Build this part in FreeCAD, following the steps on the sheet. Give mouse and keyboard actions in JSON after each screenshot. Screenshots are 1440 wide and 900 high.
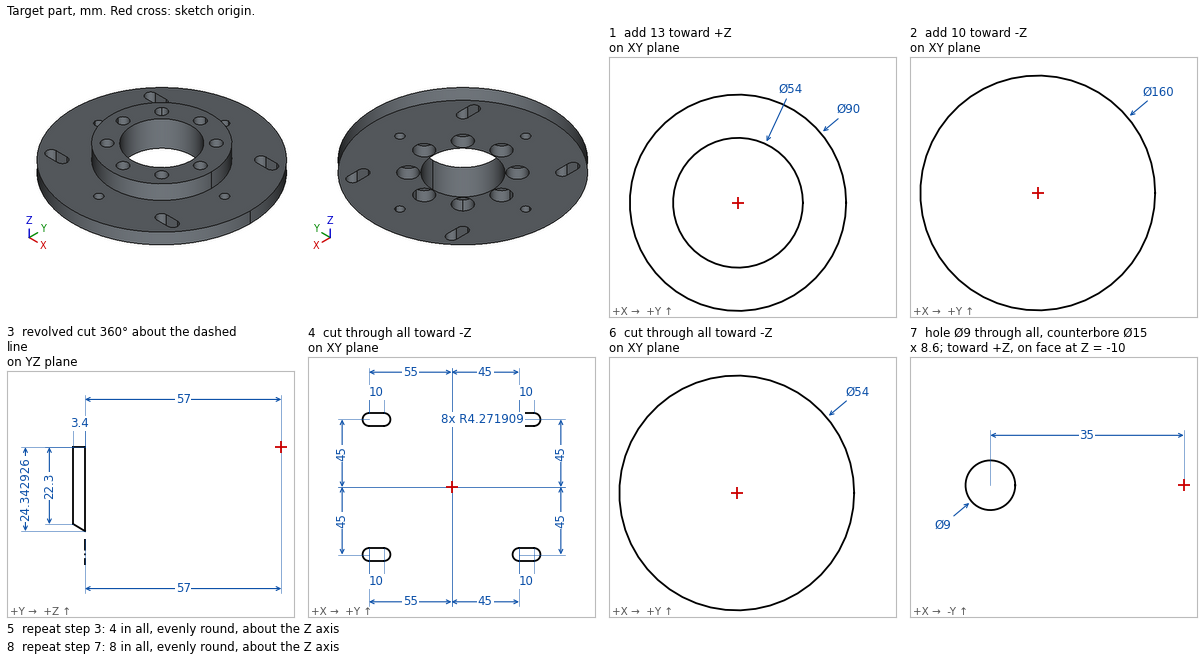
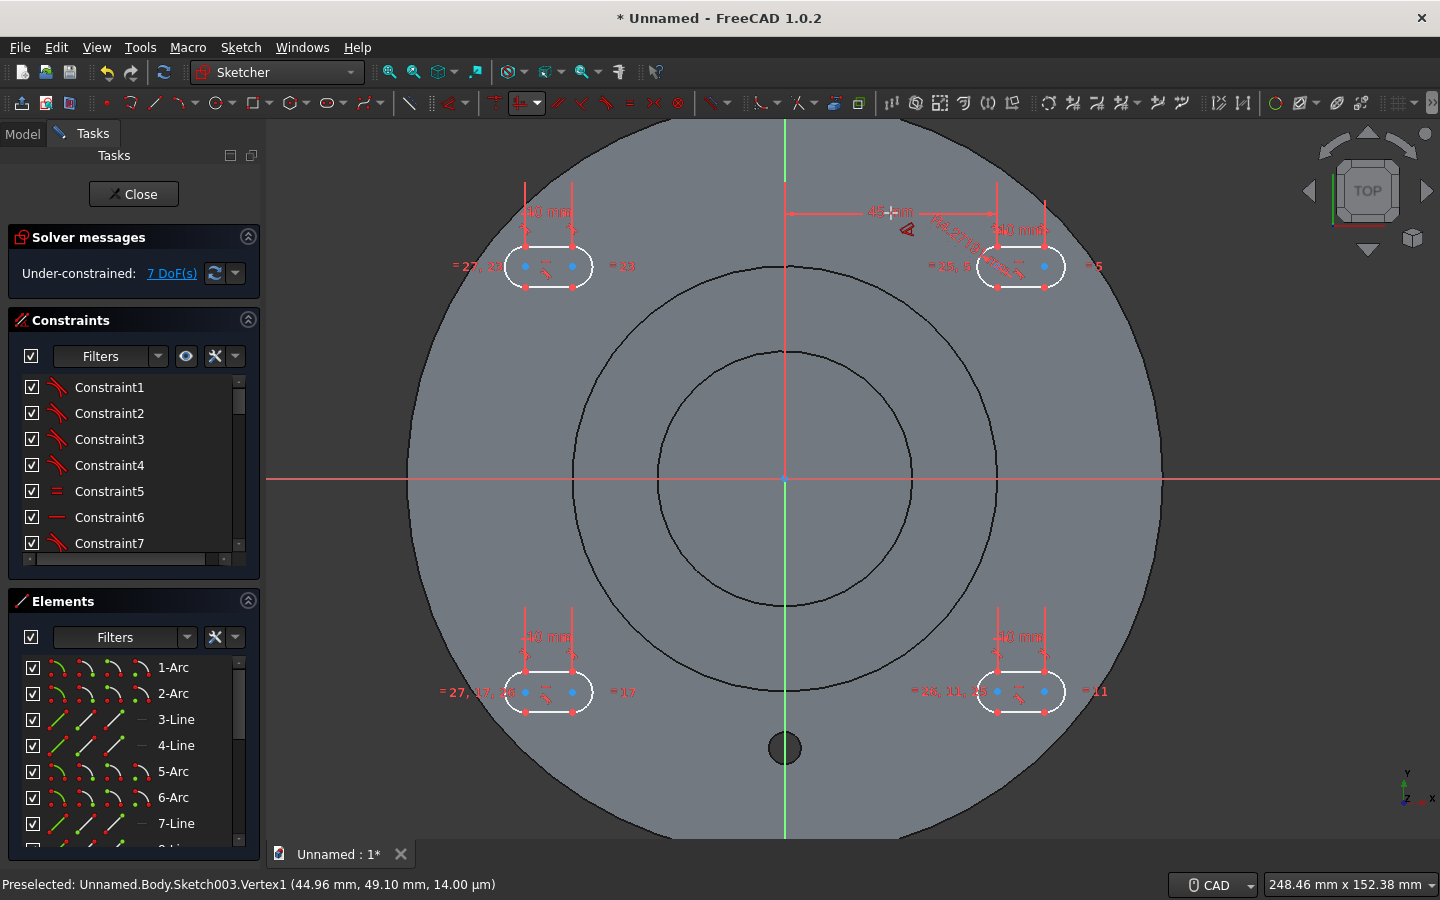
{"action": "left_click", "coordinate": [998, 672]}
{"action": "left_click", "coordinate": [891, 706]}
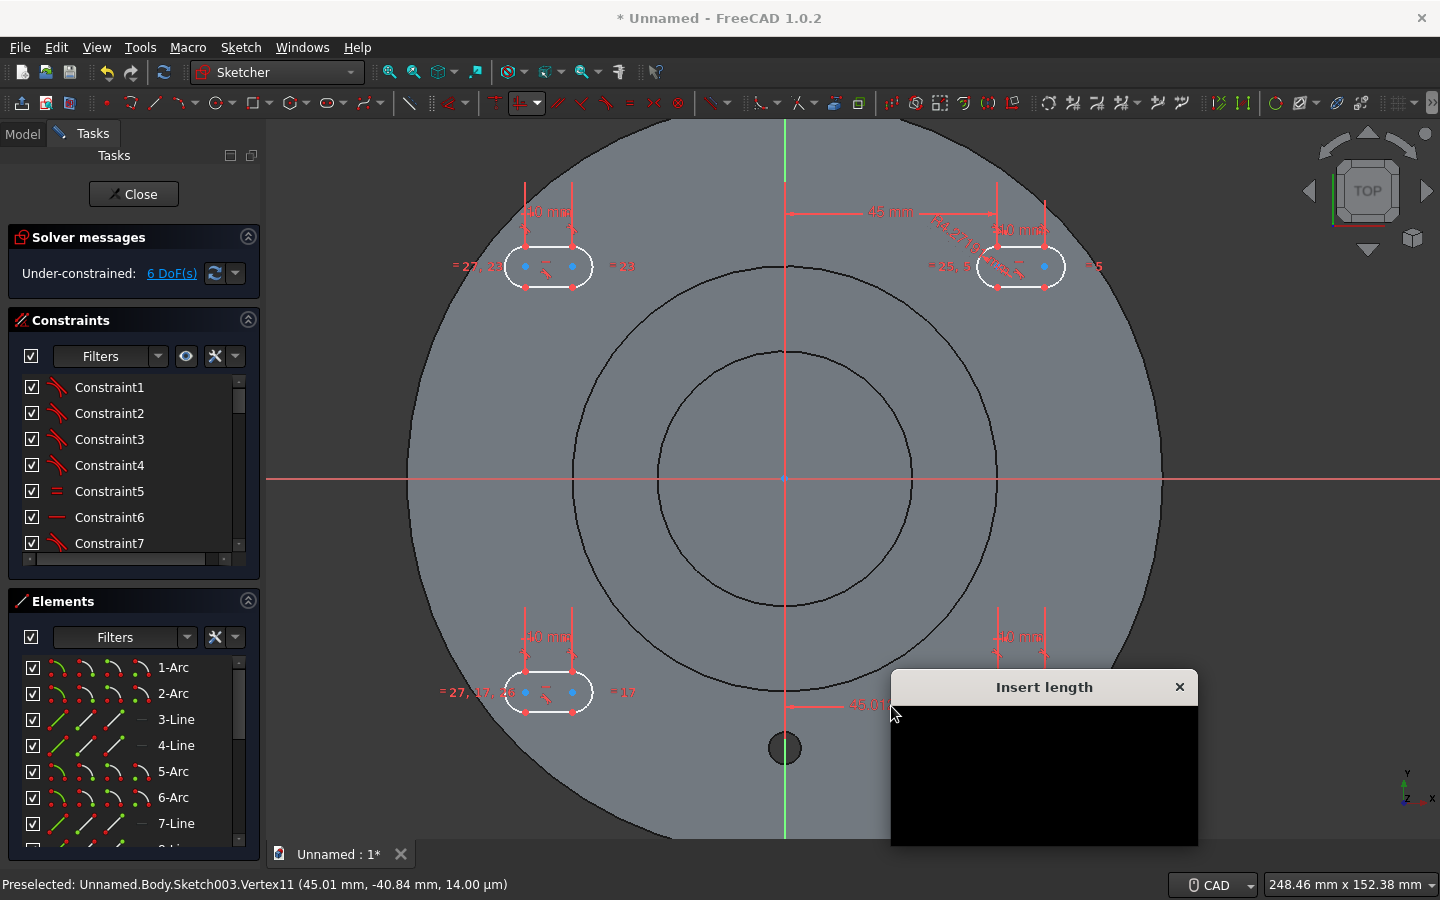
{"action": "type", "text": "45"}
{"action": "key", "text": "Return"}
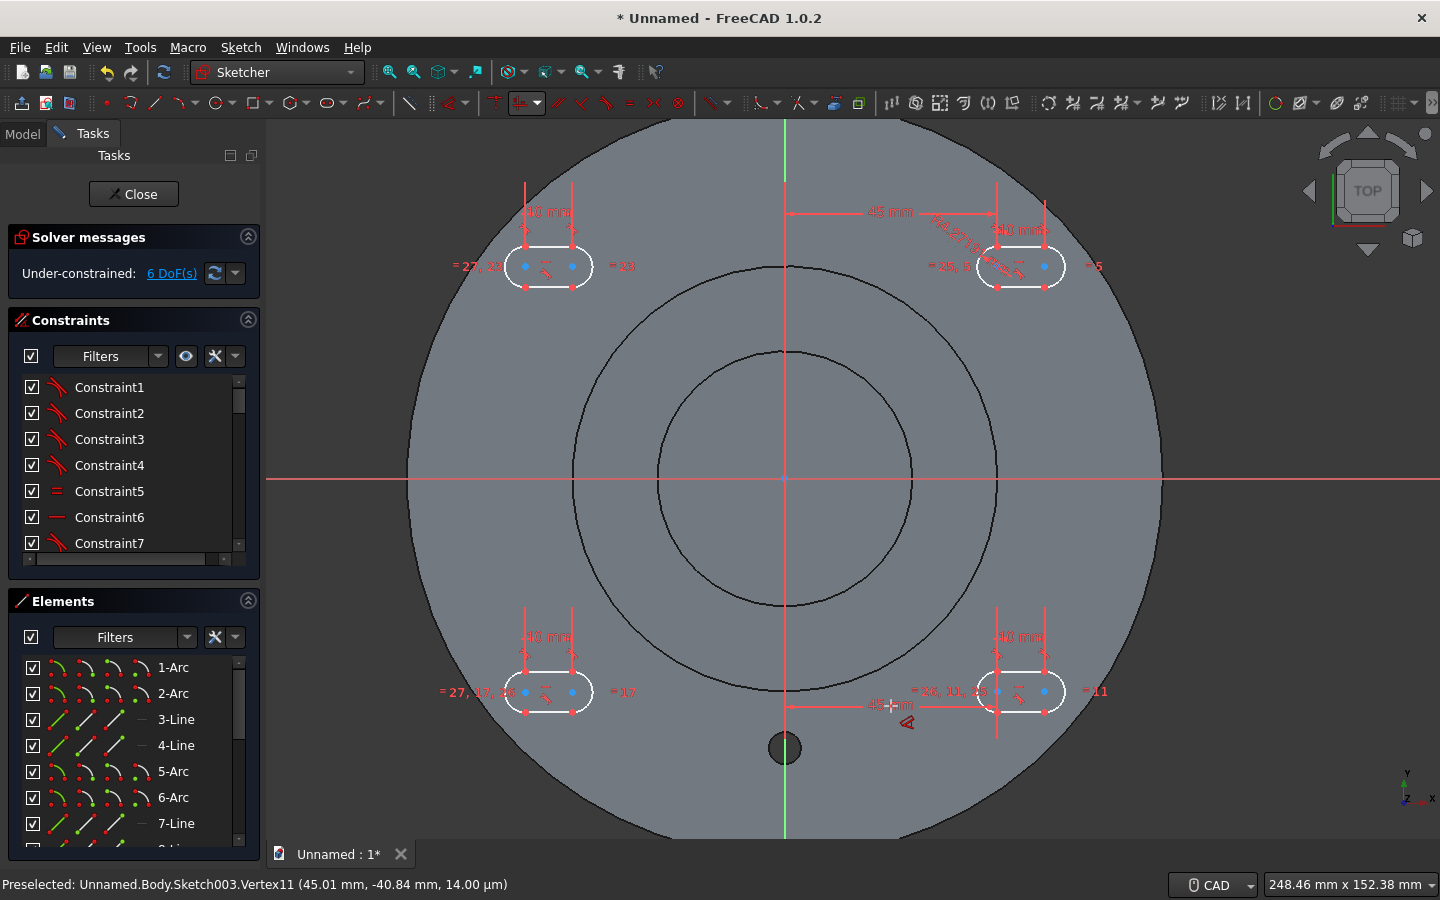
{"action": "left_click", "coordinate": [525, 672]}
{"action": "left_click", "coordinate": [655, 706]}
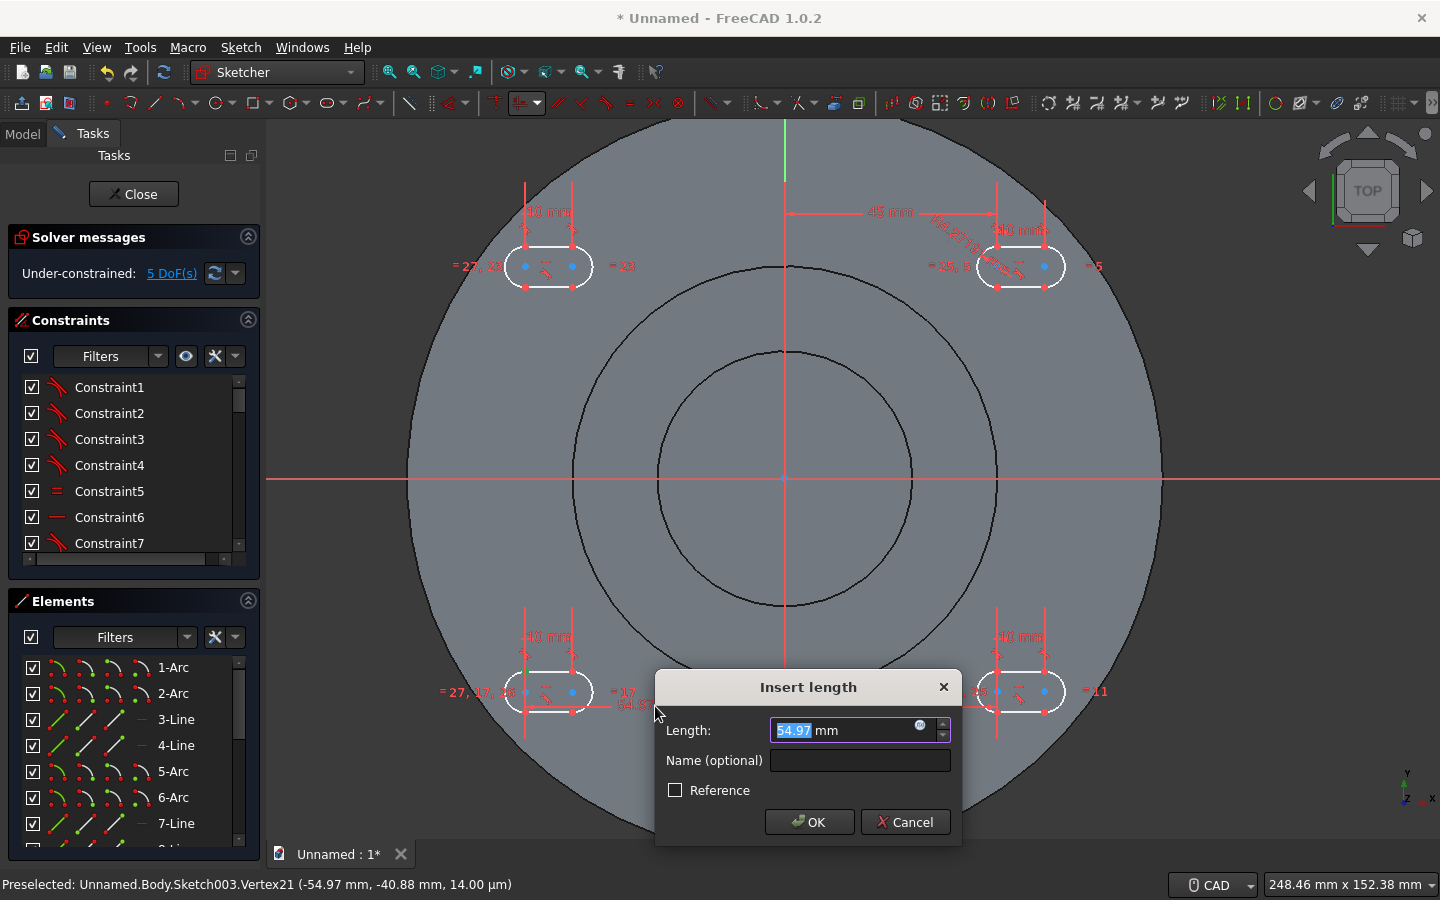
{"action": "type", "text": "55"}
{"action": "key", "text": "Return"}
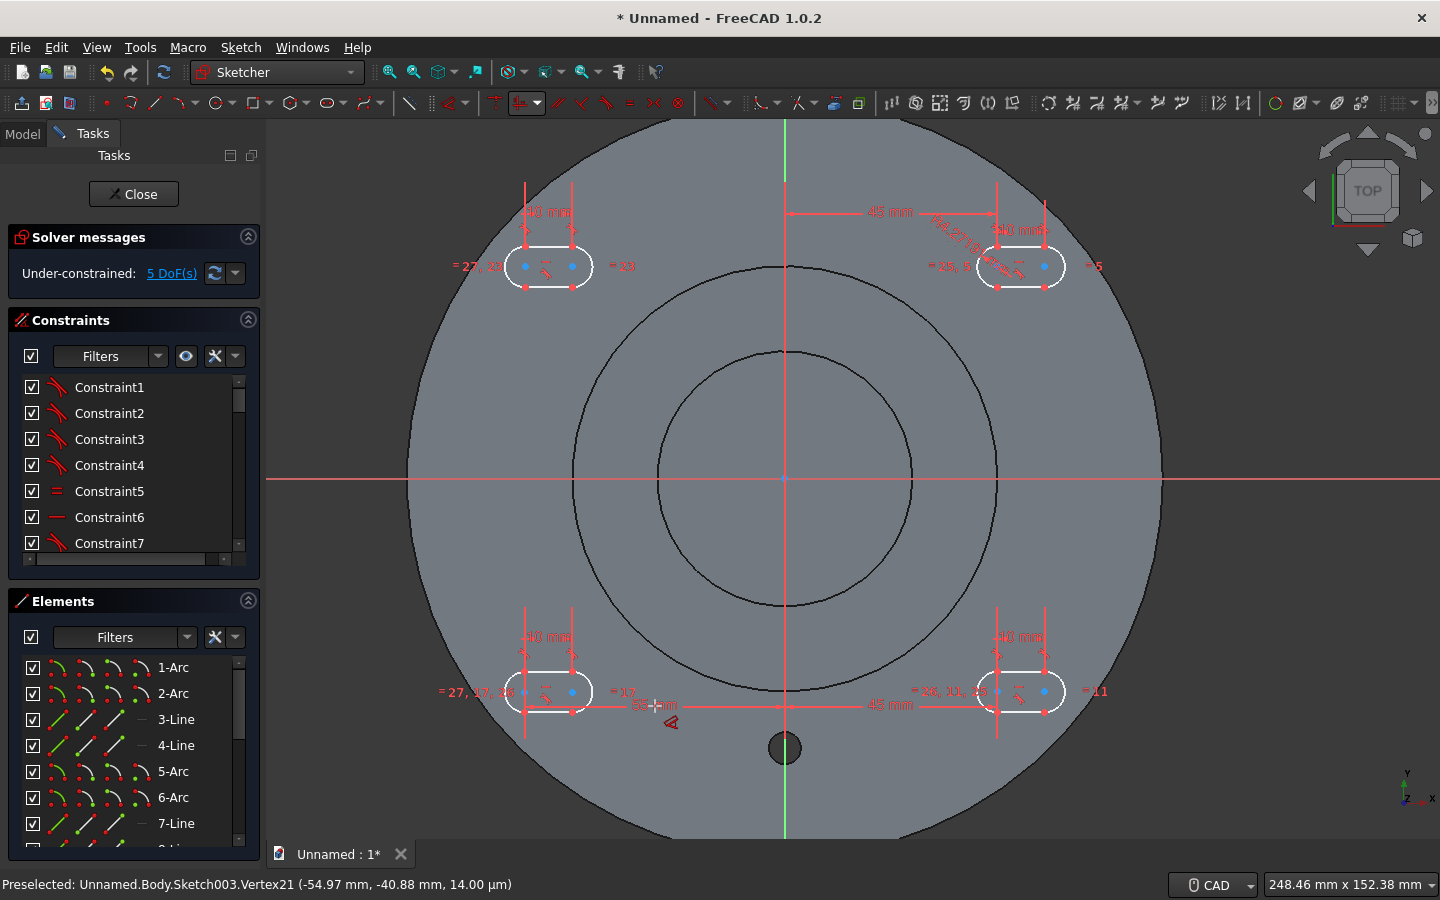
{"action": "left_click", "coordinate": [525, 247]}
{"action": "left_click", "coordinate": [655, 213]}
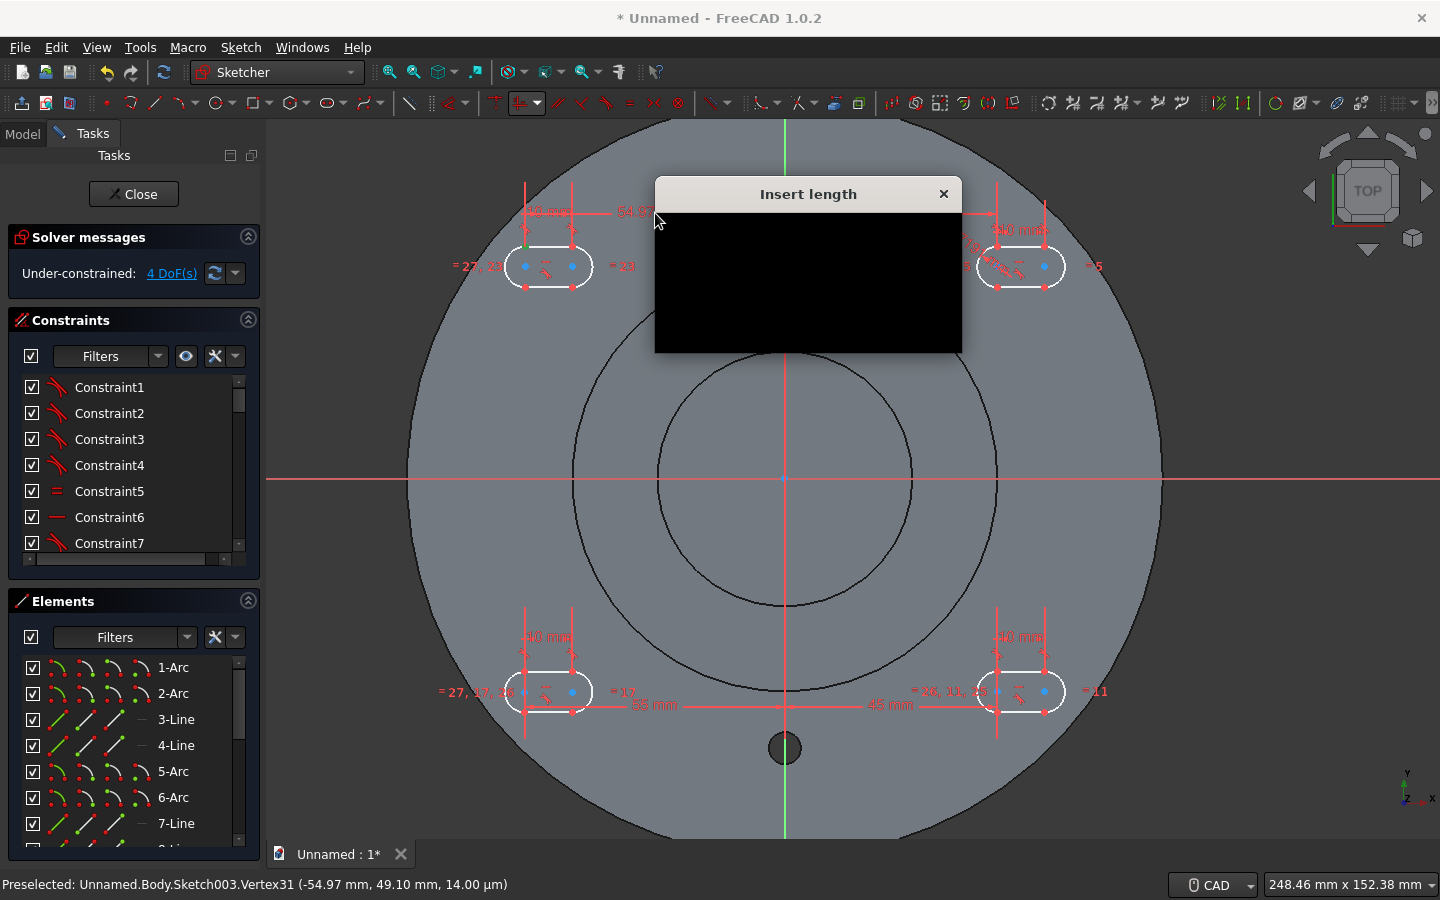
{"action": "type", "text": "55"}
{"action": "key", "text": "Return"}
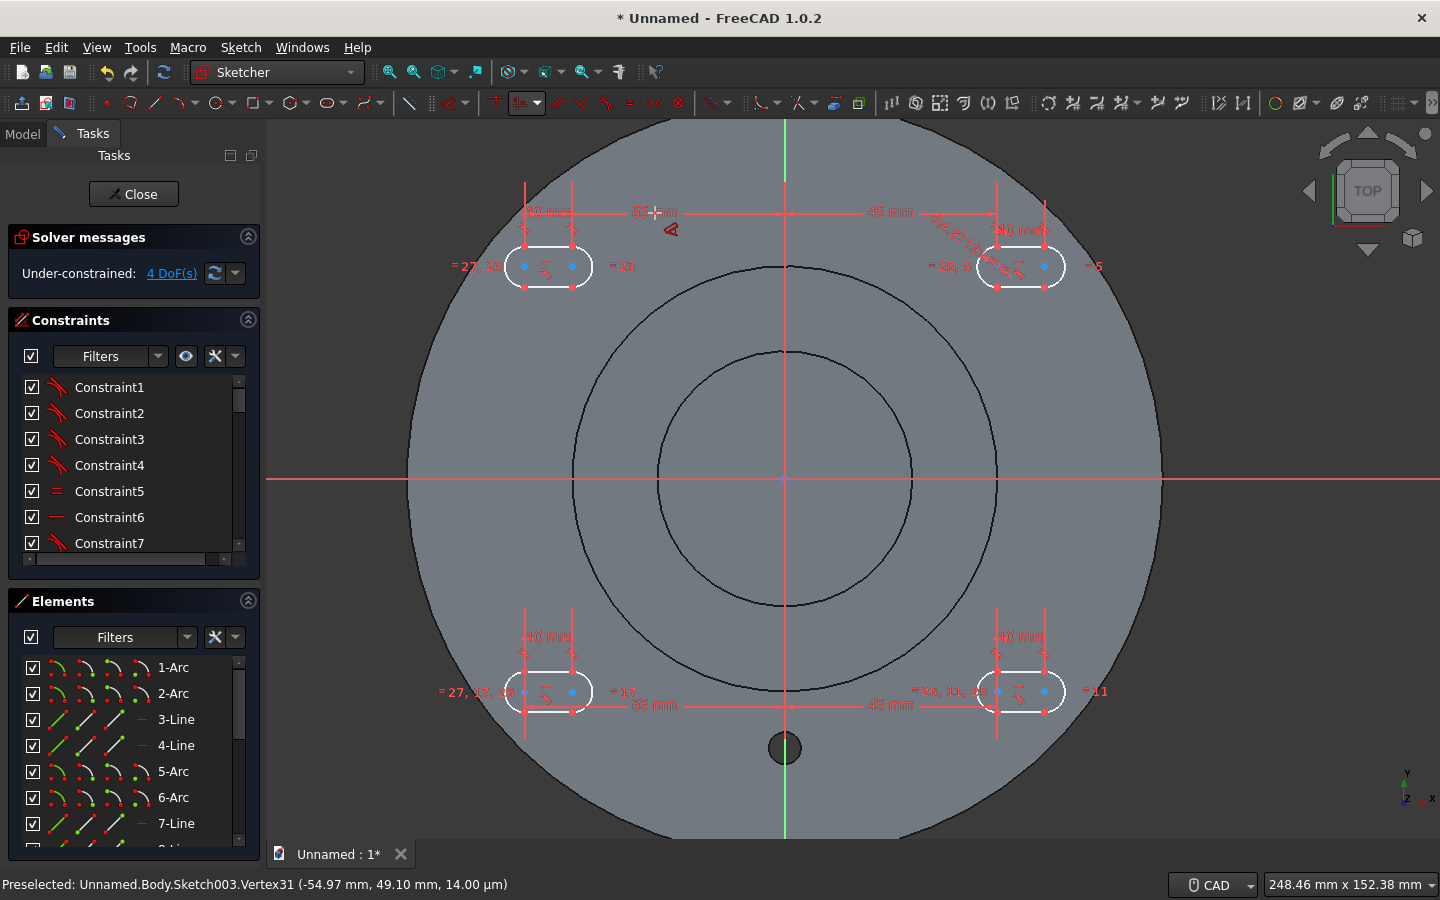
{"action": "left_click", "coordinate": [997, 267]}
{"action": "left_click", "coordinate": [1031, 373]}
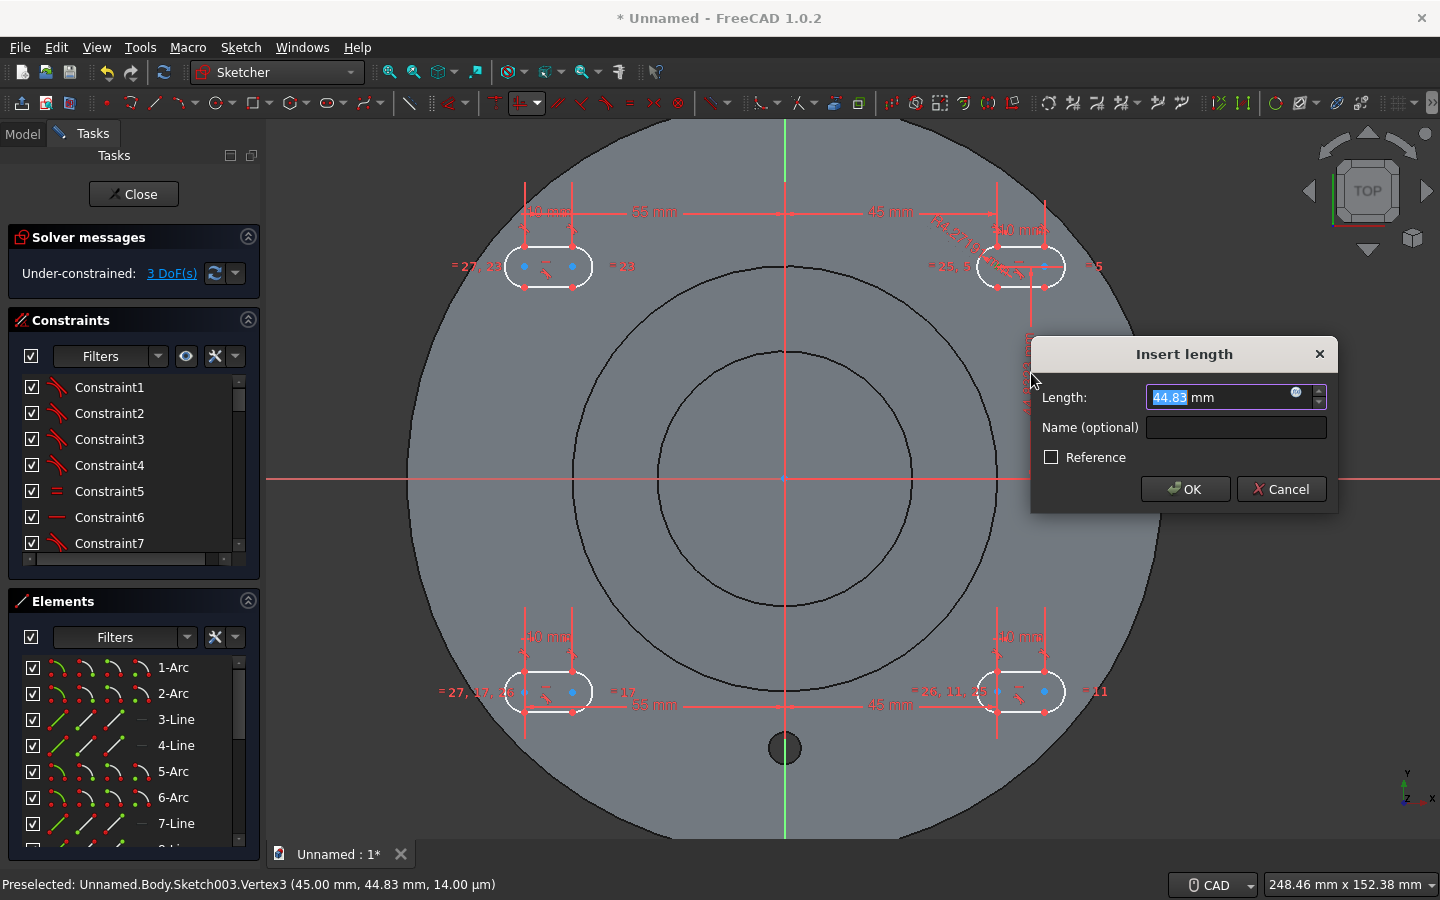
{"action": "type", "text": "45"}
{"action": "key", "text": "Return"}